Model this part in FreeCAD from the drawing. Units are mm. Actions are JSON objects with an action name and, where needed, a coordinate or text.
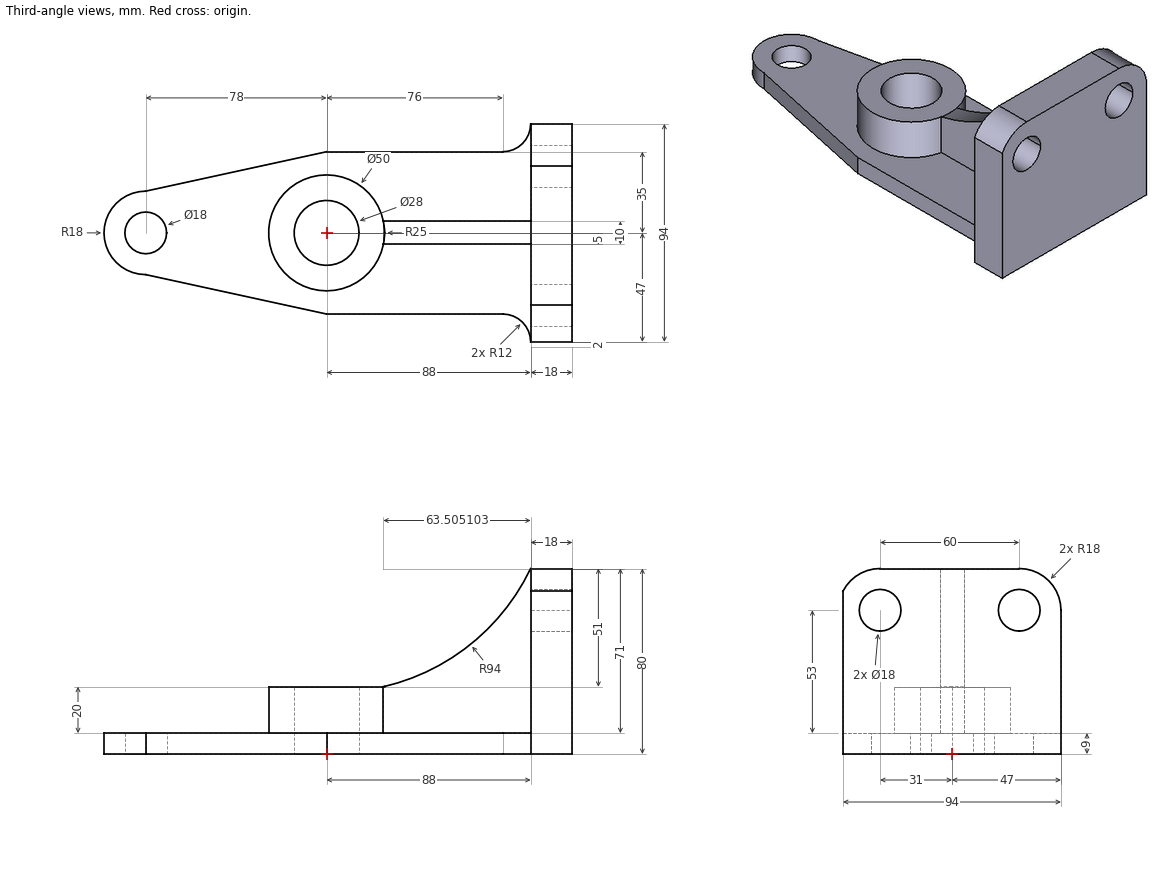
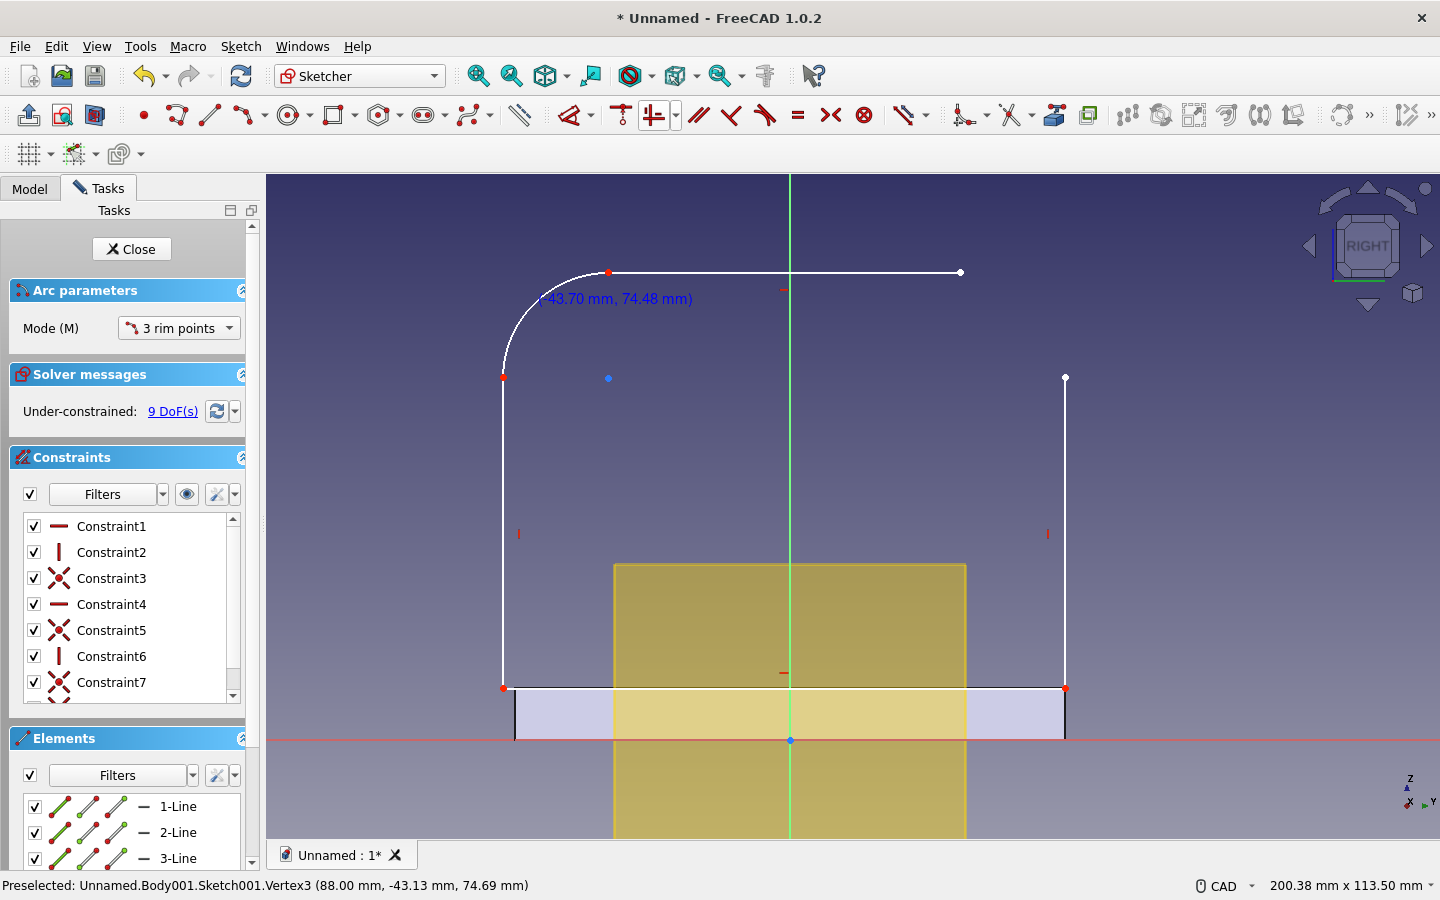
{"action": "left_click", "coordinate": [1065, 378]}
{"action": "left_click", "coordinate": [960, 273]}
{"action": "left_click", "coordinate": [1035, 303]}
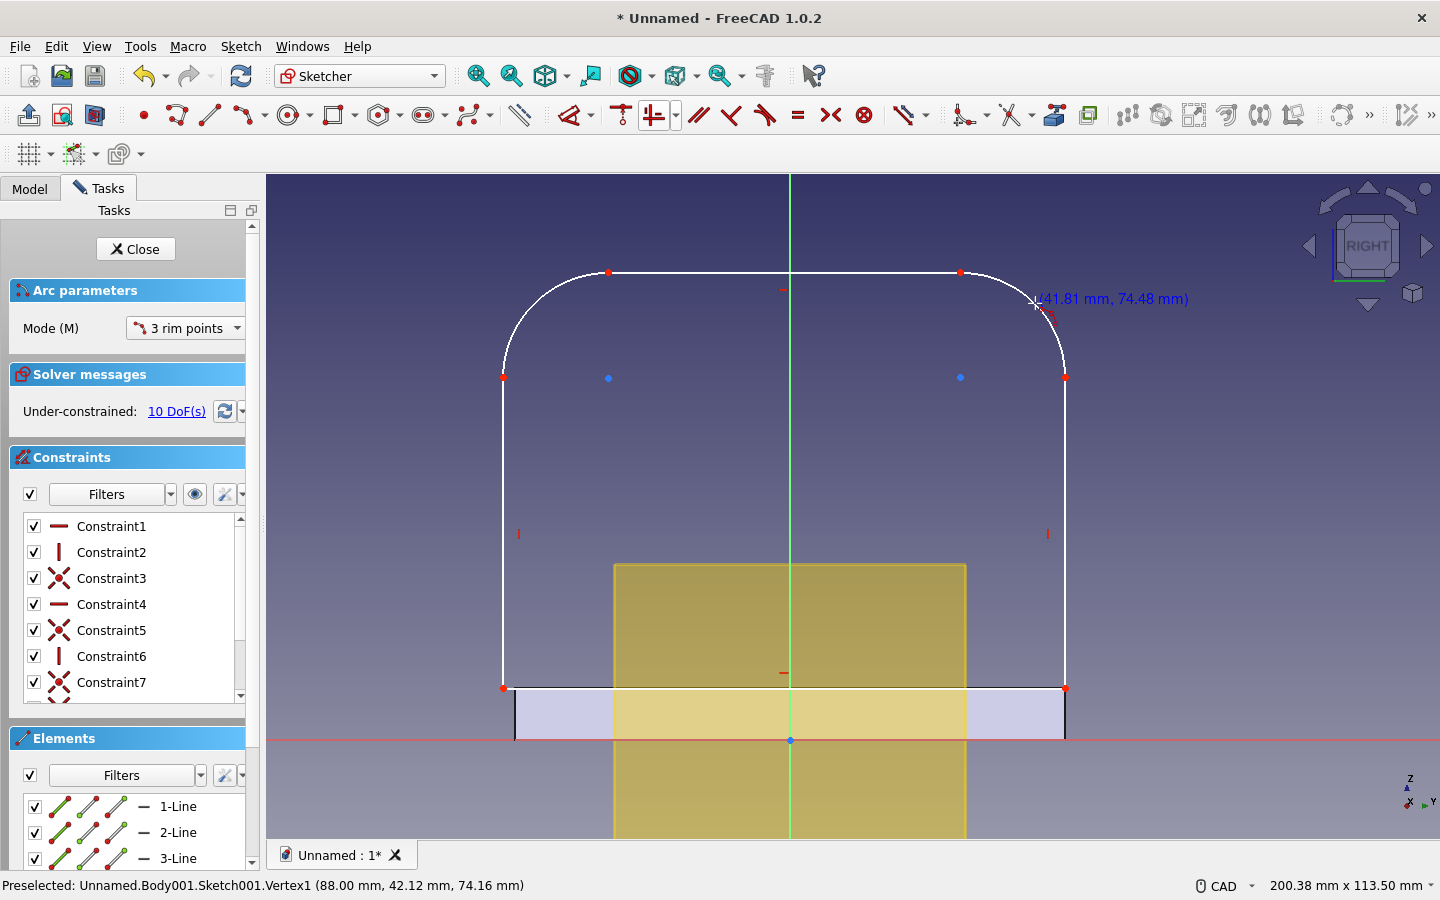
{"action": "left_click", "coordinate": [288, 116]}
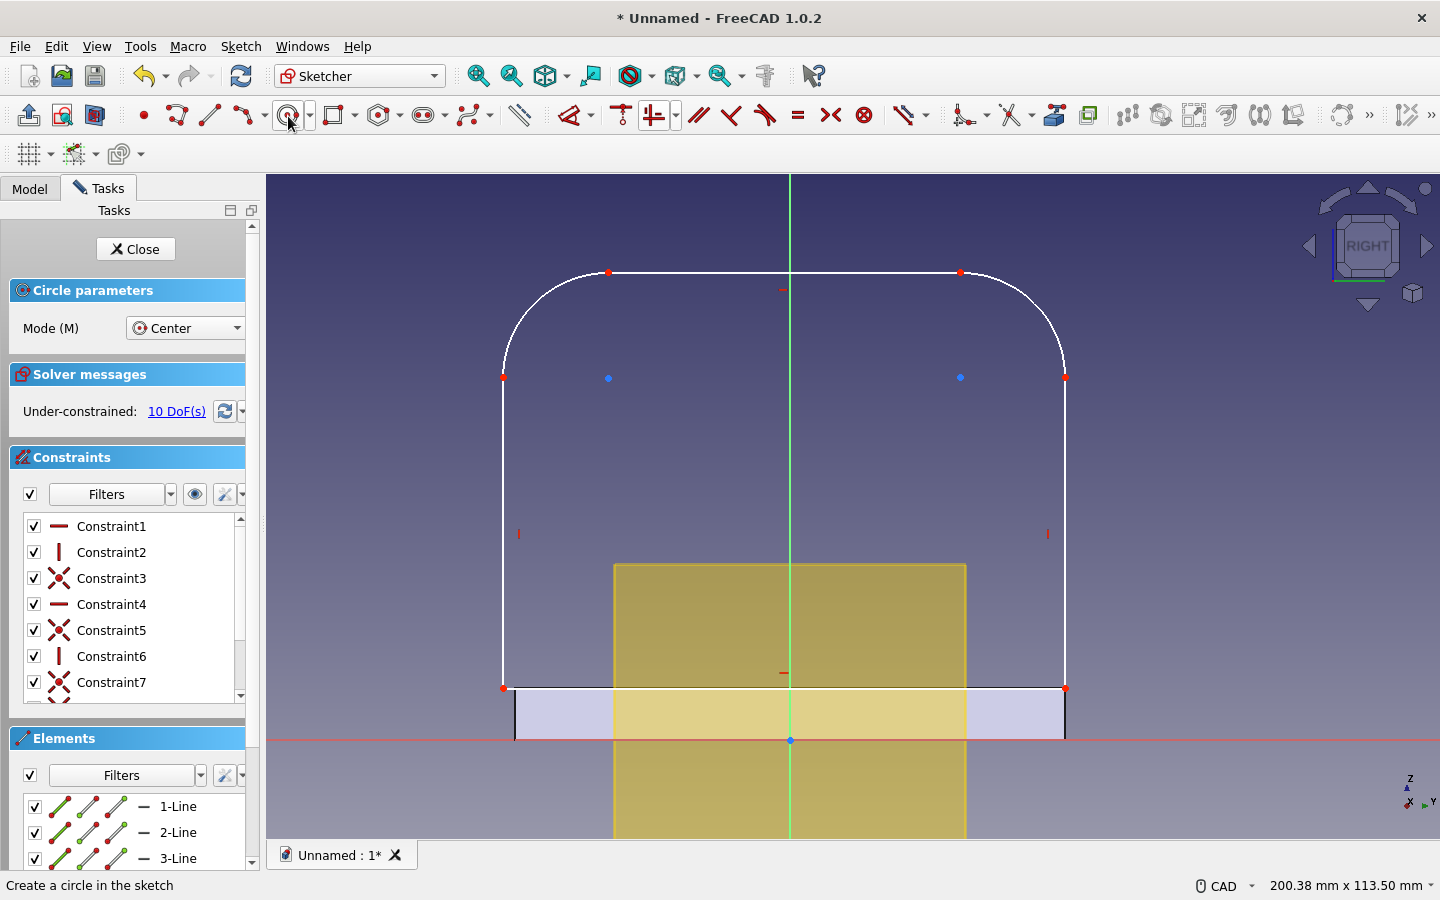
{"action": "left_click", "coordinate": [608, 377]}
{"action": "left_click", "coordinate": [646, 340]}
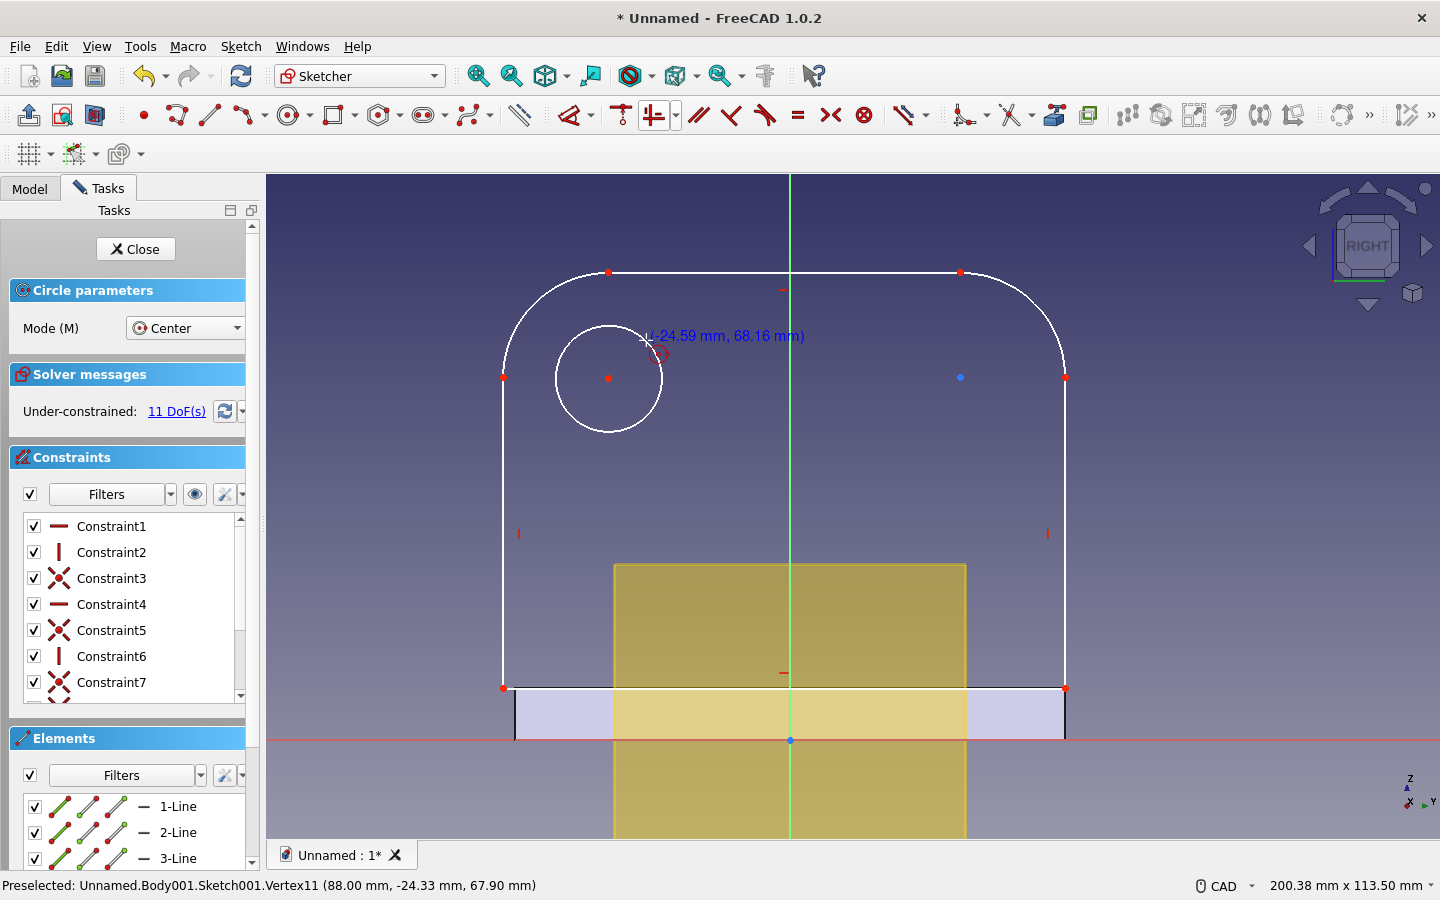
{"action": "left_click", "coordinate": [960, 377]}
{"action": "left_click", "coordinate": [997, 340]}
{"action": "key", "text": "Escape"}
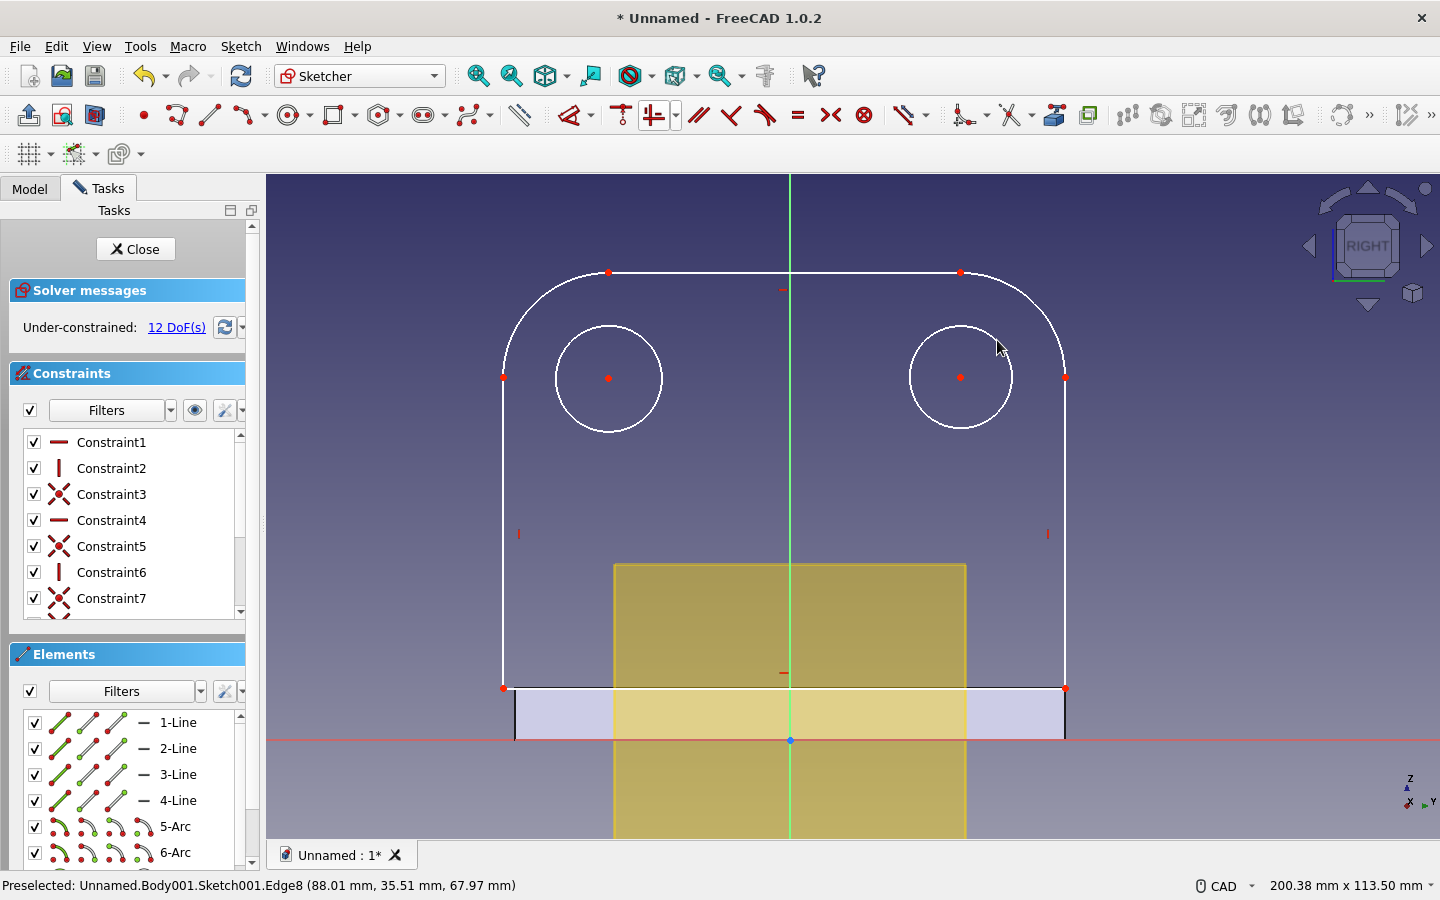
{"action": "left_click", "coordinate": [854, 273]}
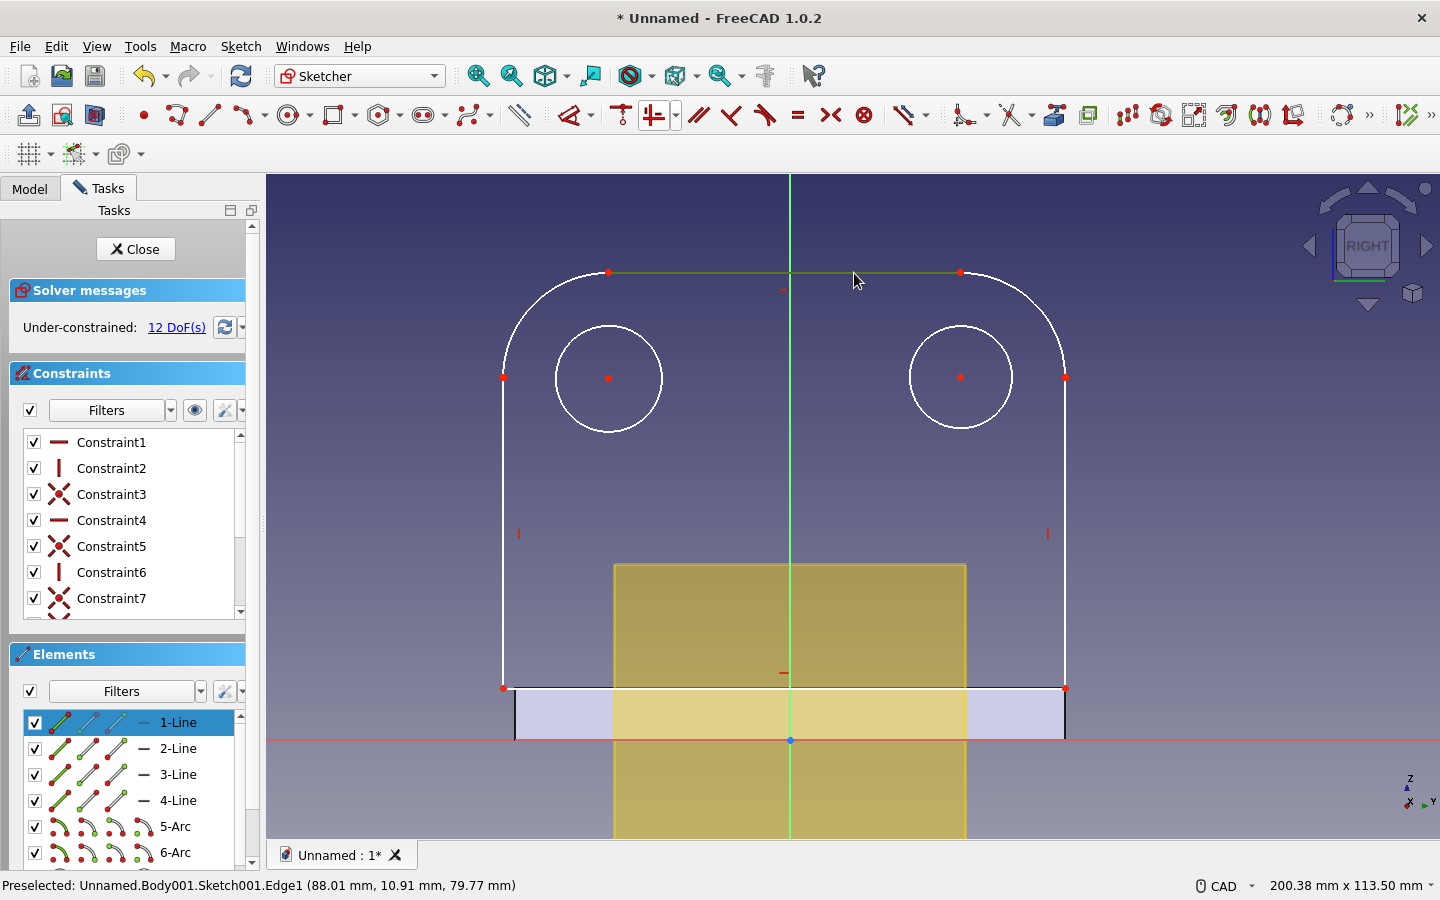
{"action": "left_click", "coordinate": [560, 285]}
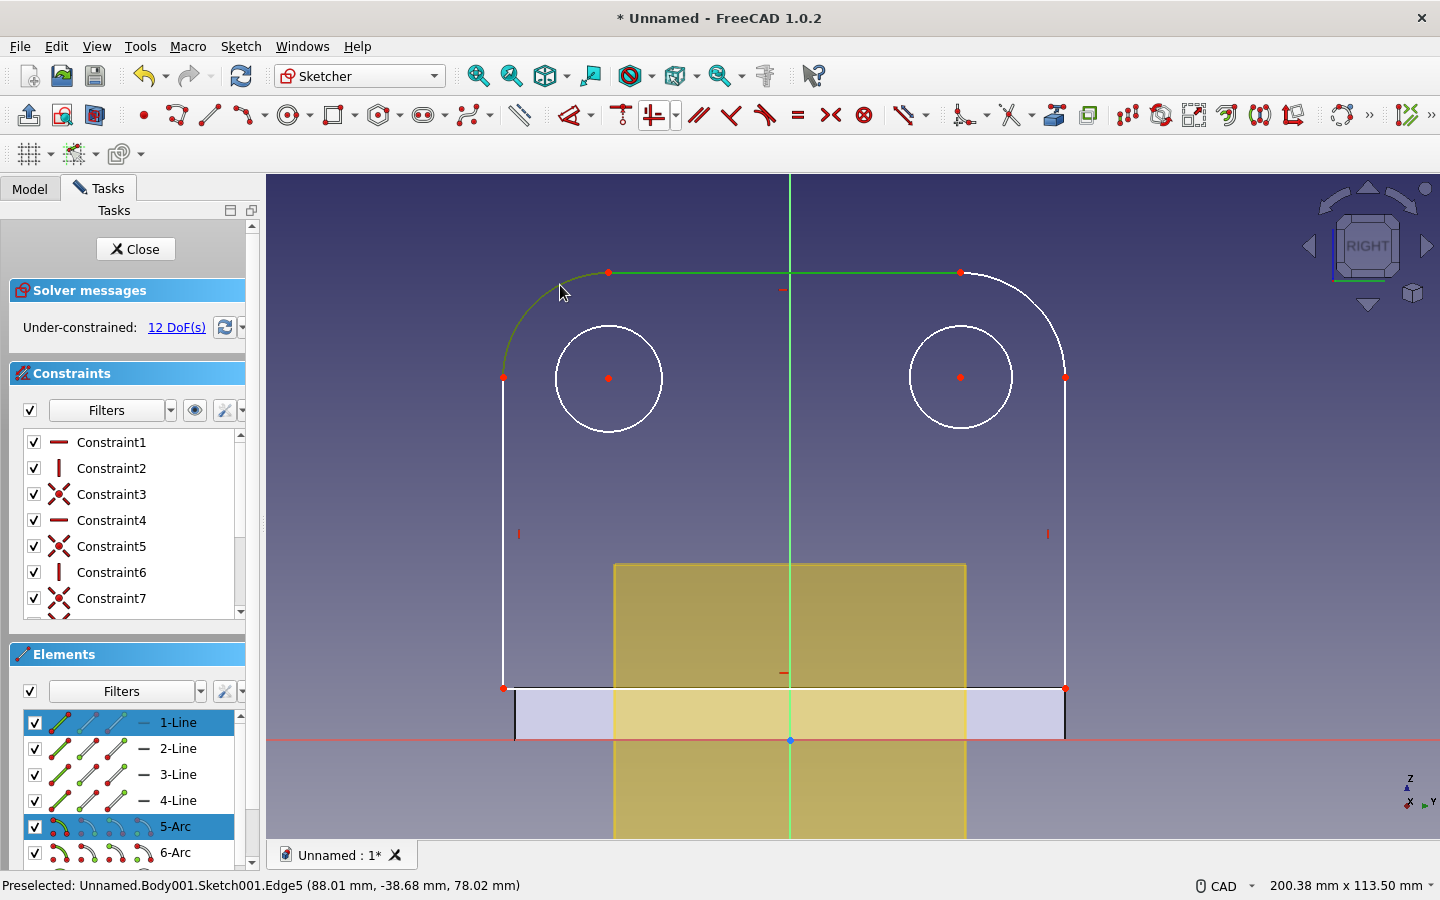
{"action": "left_click", "coordinate": [765, 116]}